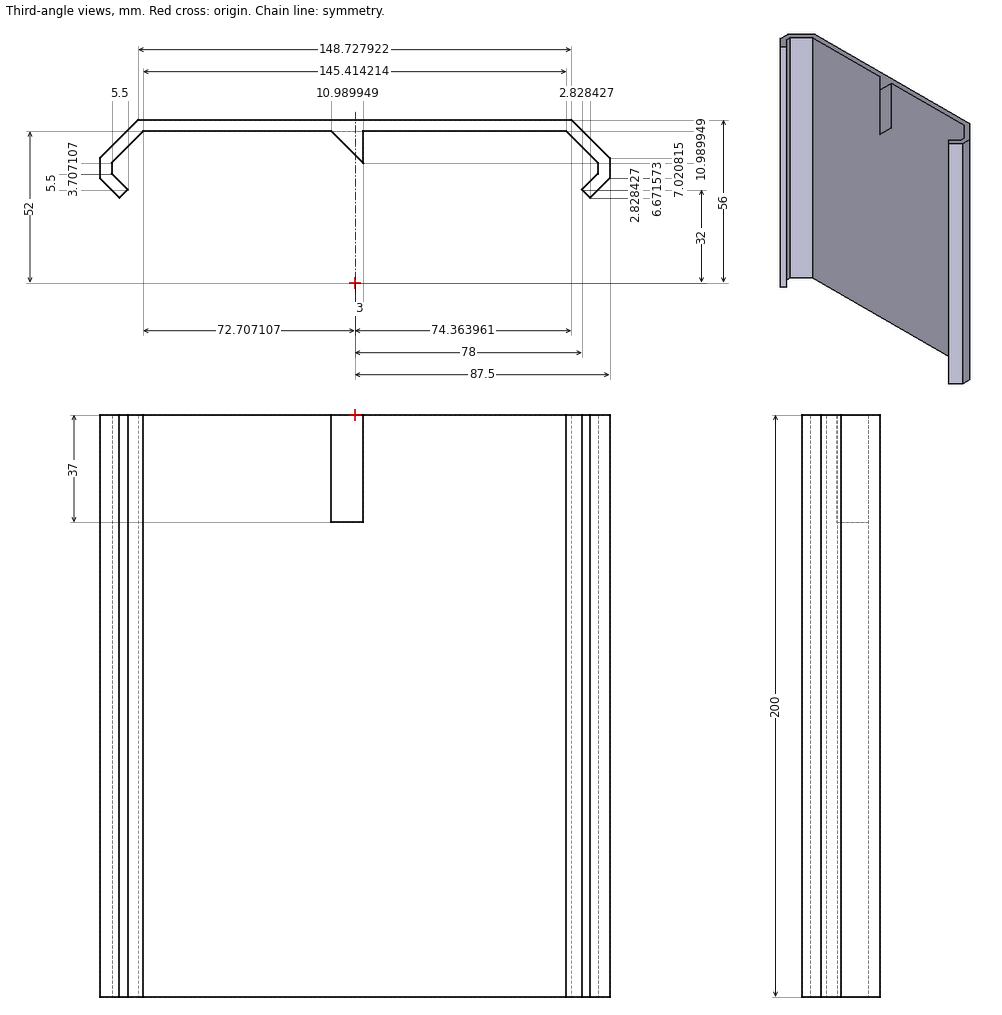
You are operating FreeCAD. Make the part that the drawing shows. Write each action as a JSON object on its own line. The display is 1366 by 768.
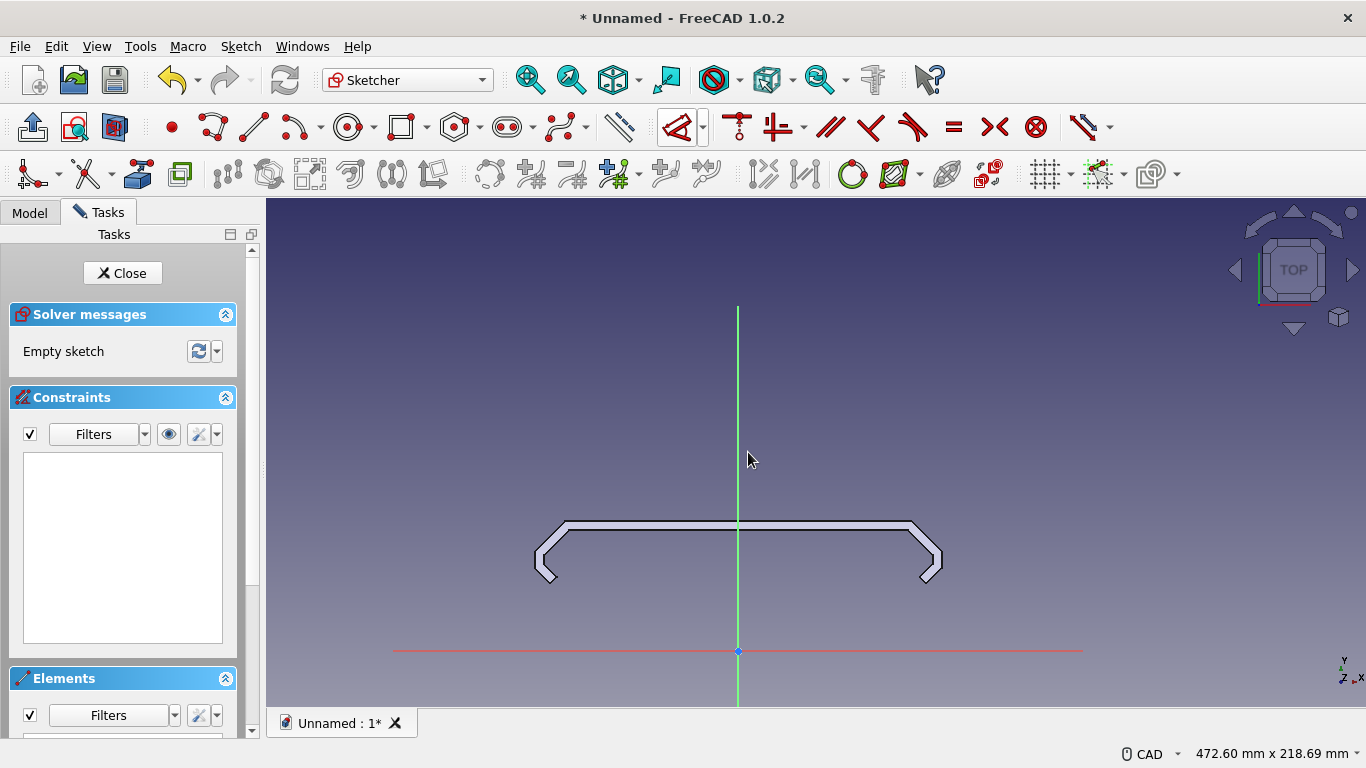
{"action": "scroll", "coordinate": [731, 550], "scroll_direction": "up", "scroll_amount": 13}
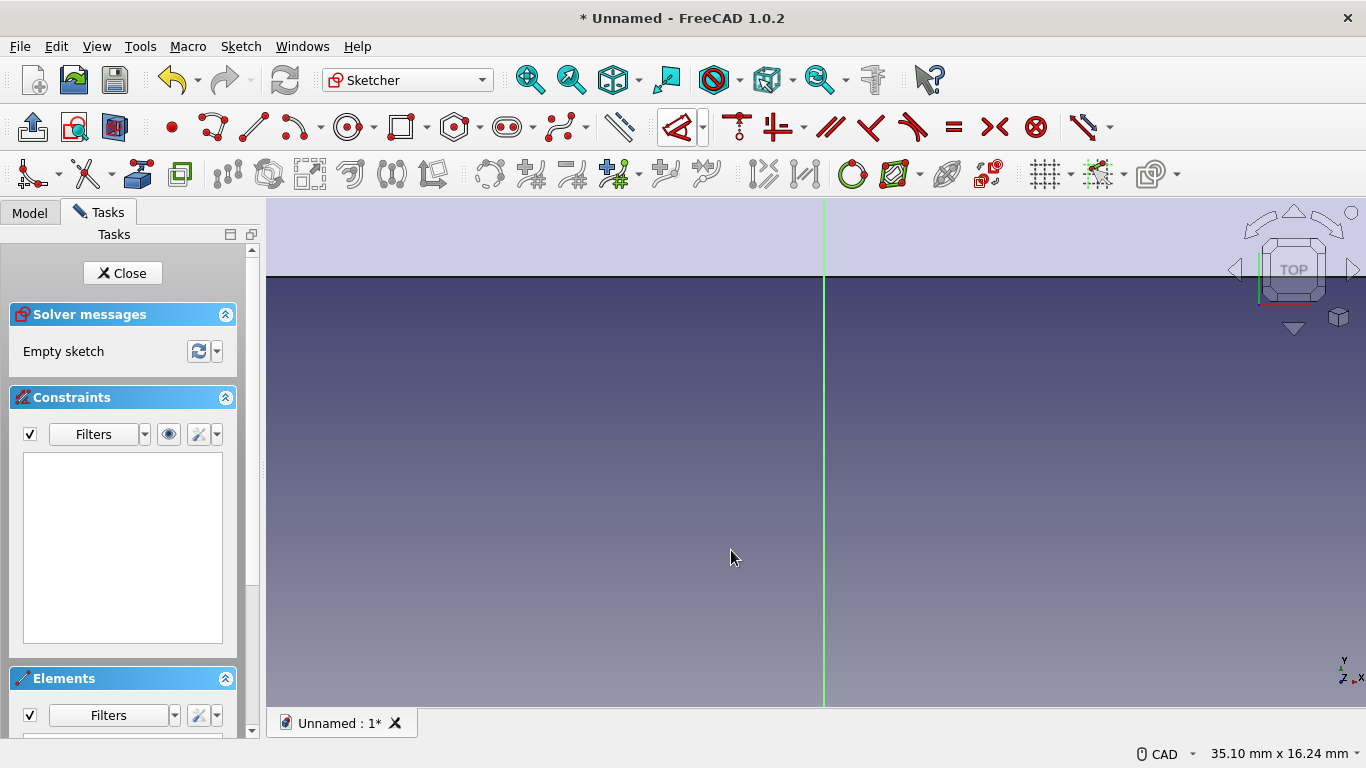
{"action": "left_click", "coordinate": [213, 128]}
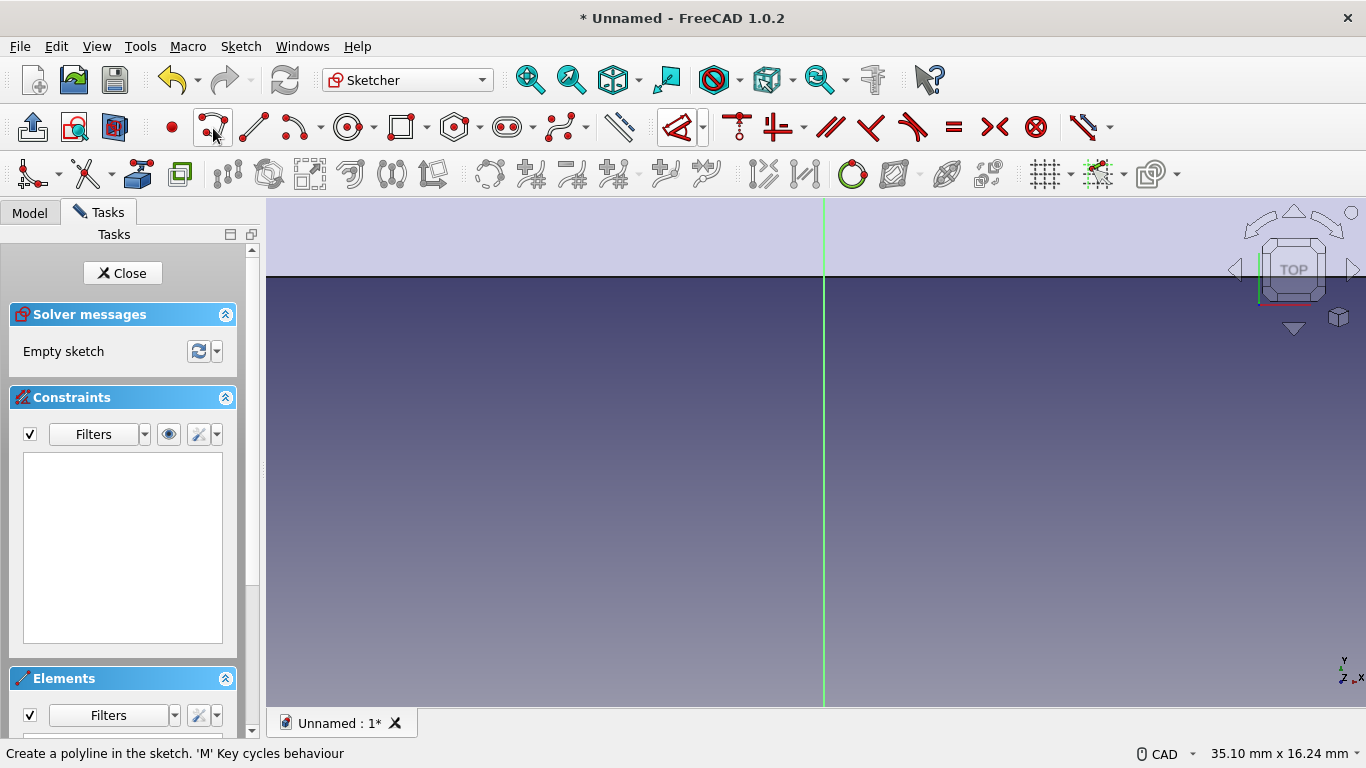
{"action": "left_click", "coordinate": [918, 621]}
{"action": "left_click", "coordinate": [918, 277]}
{"action": "left_click", "coordinate": [574, 277]}
{"action": "left_click", "coordinate": [918, 622]}
{"action": "key", "text": "Escape"}
{"action": "key", "text": "Escape"}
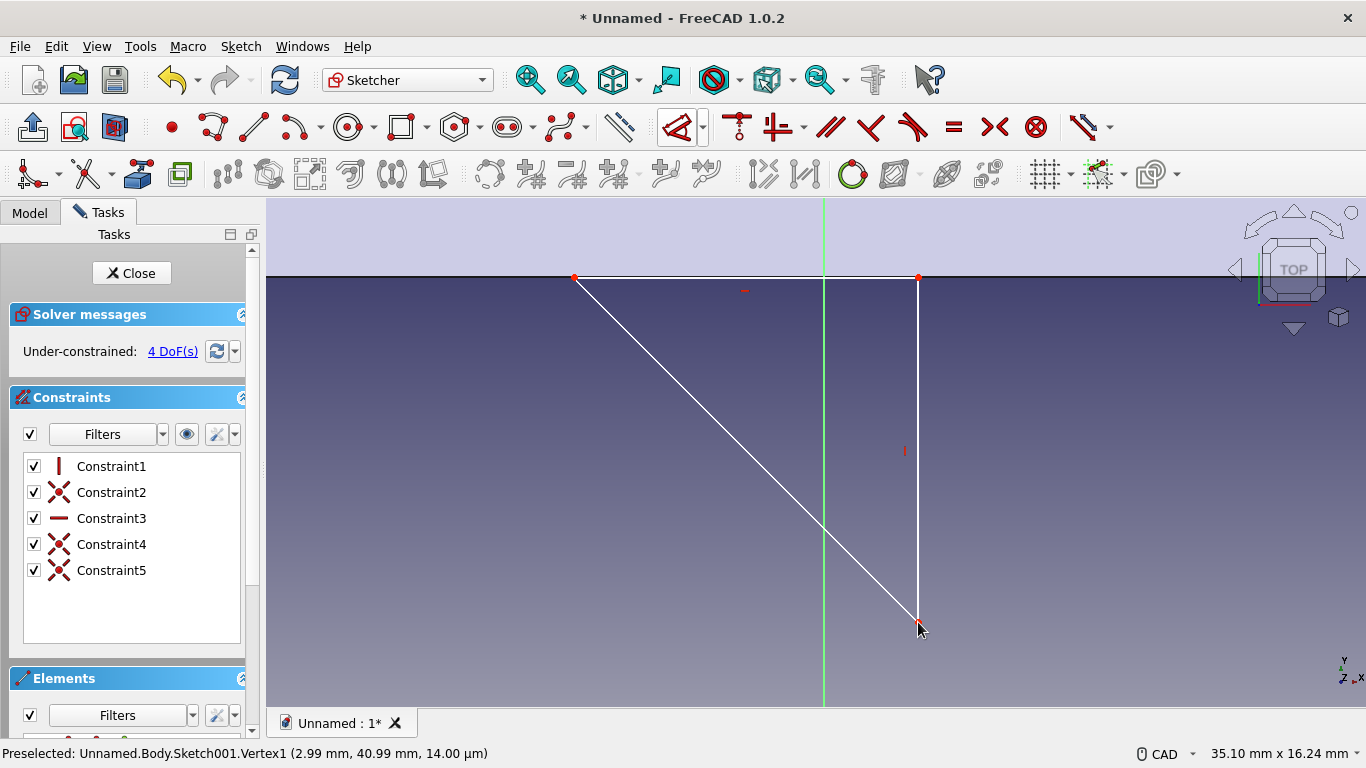
{"action": "left_click", "coordinate": [918, 622]}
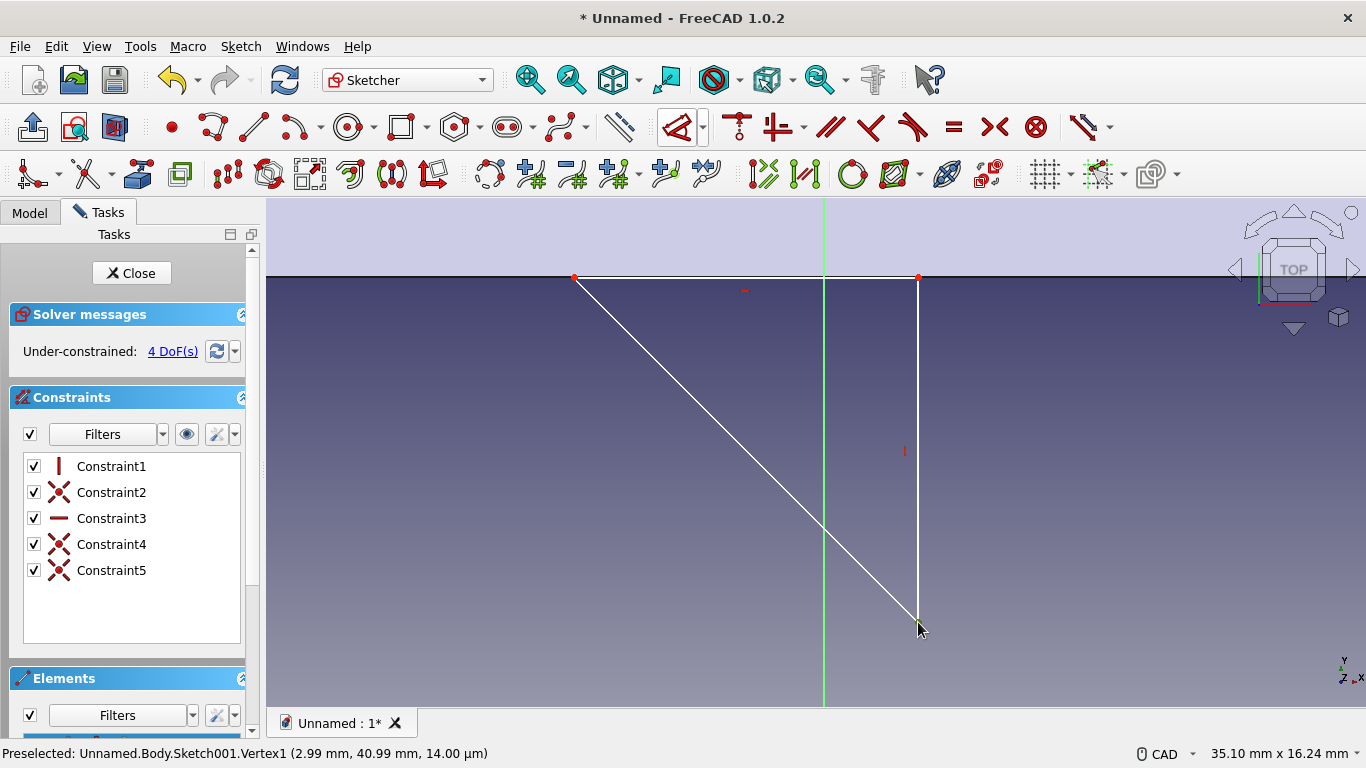
{"action": "key", "text": "l"}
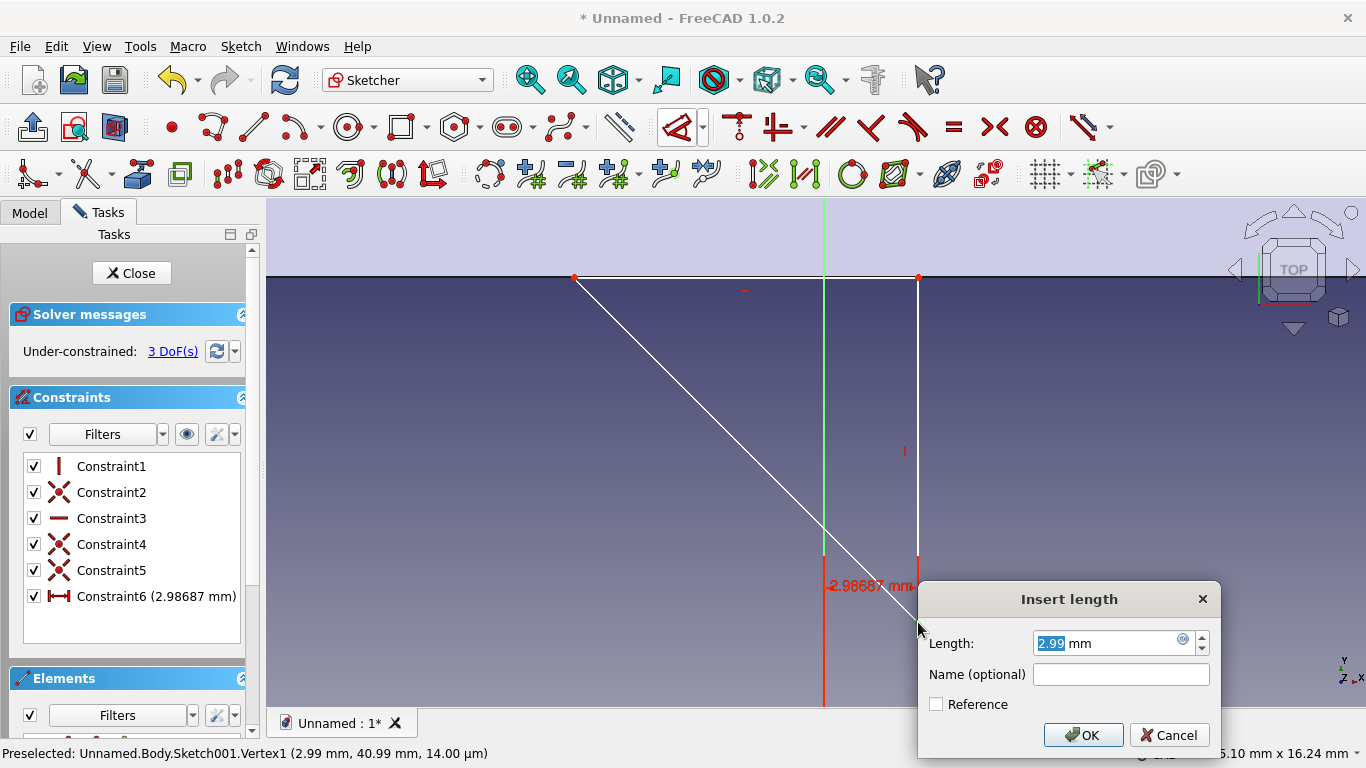
{"action": "type", "text": "3"}
{"action": "key", "text": "Return"}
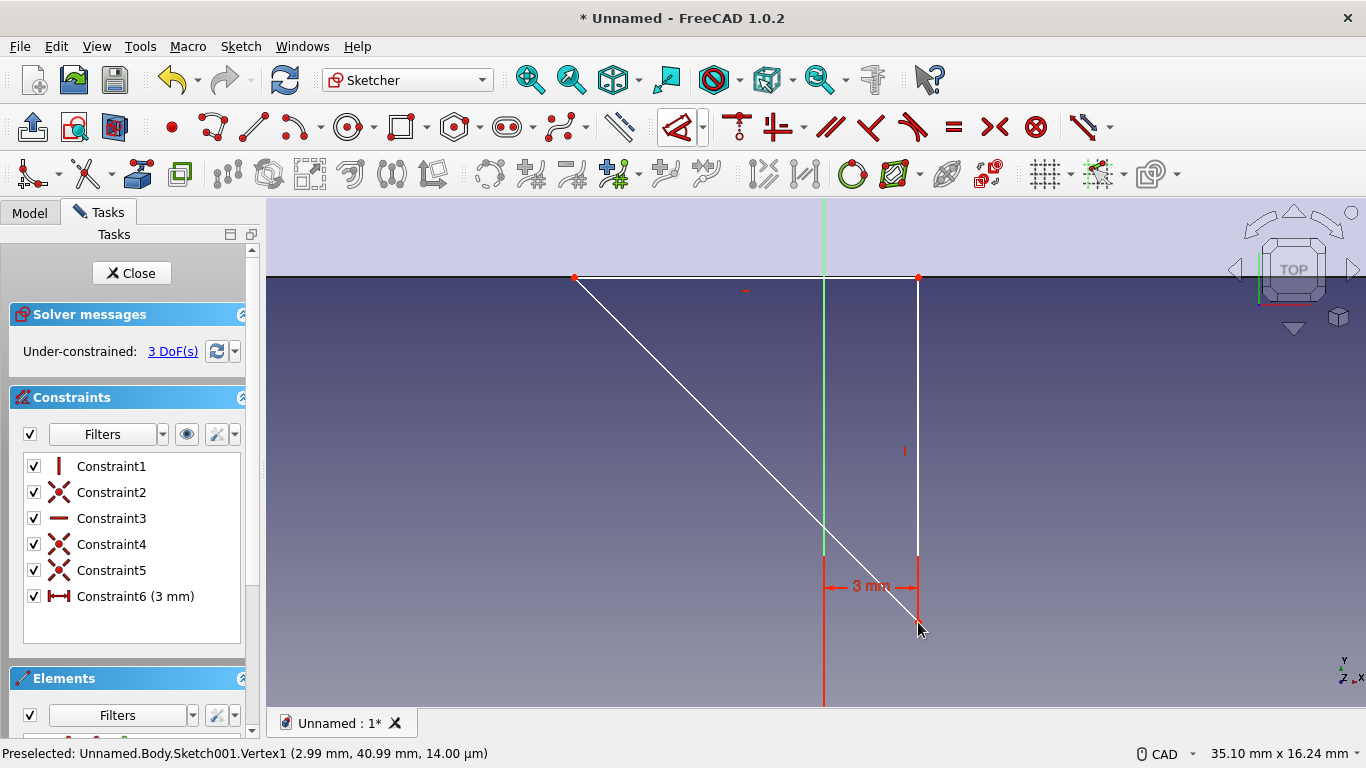
{"action": "left_click", "coordinate": [918, 278]}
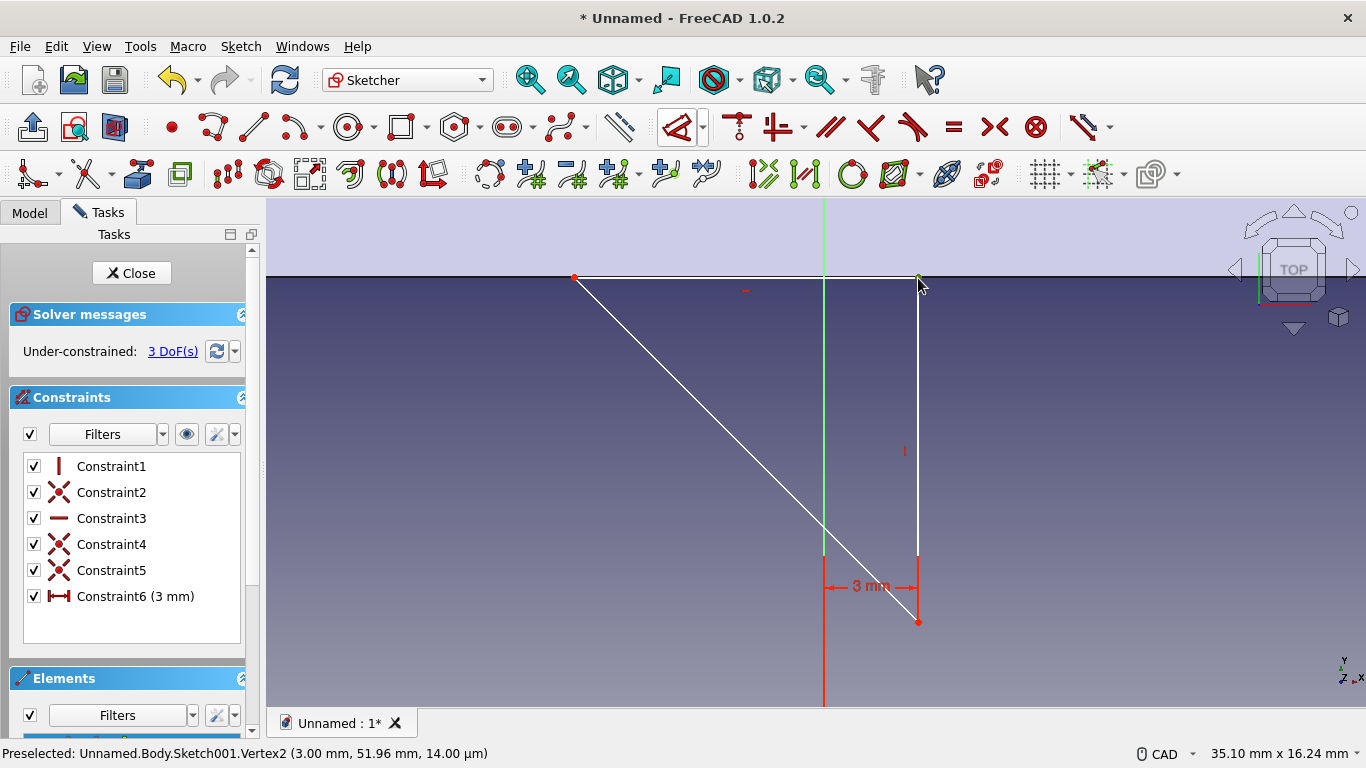
{"action": "left_click", "coordinate": [702, 128]}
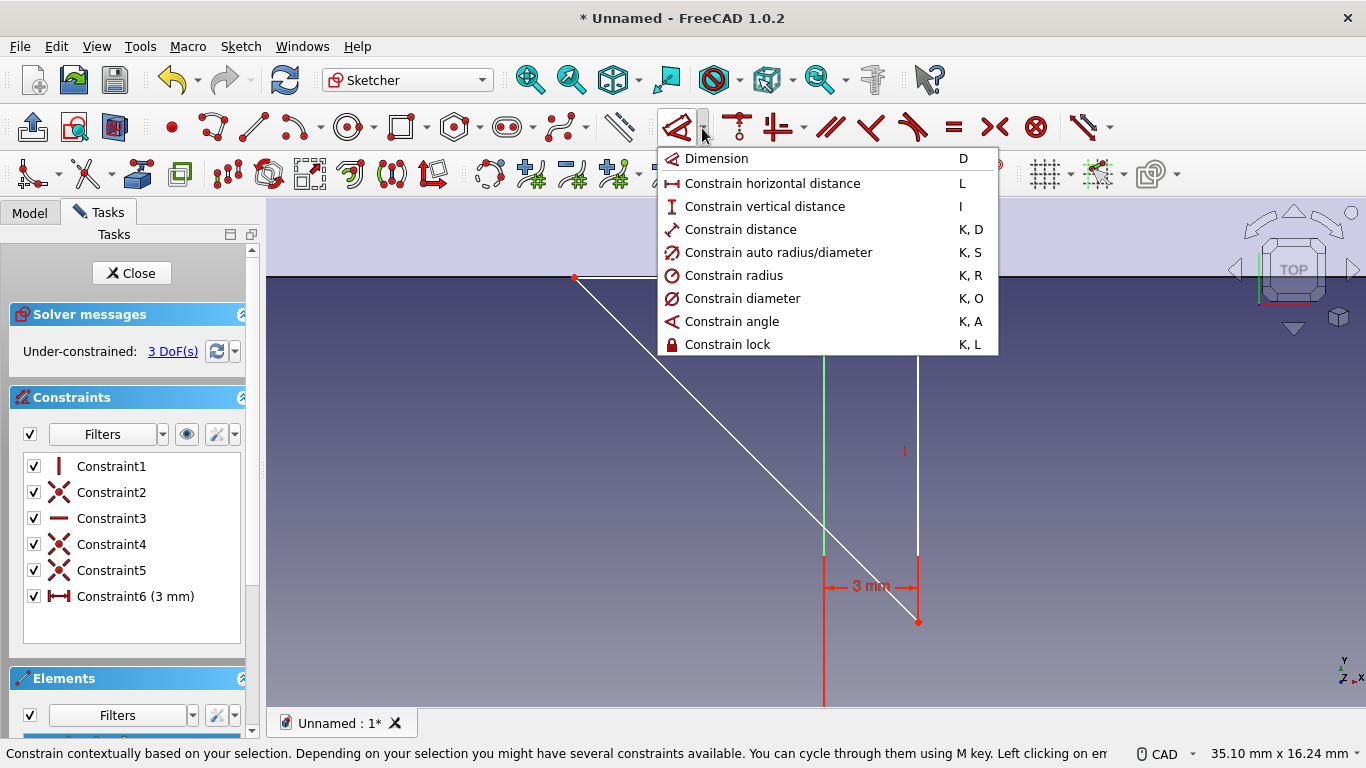
{"action": "left_click", "coordinate": [828, 206]}